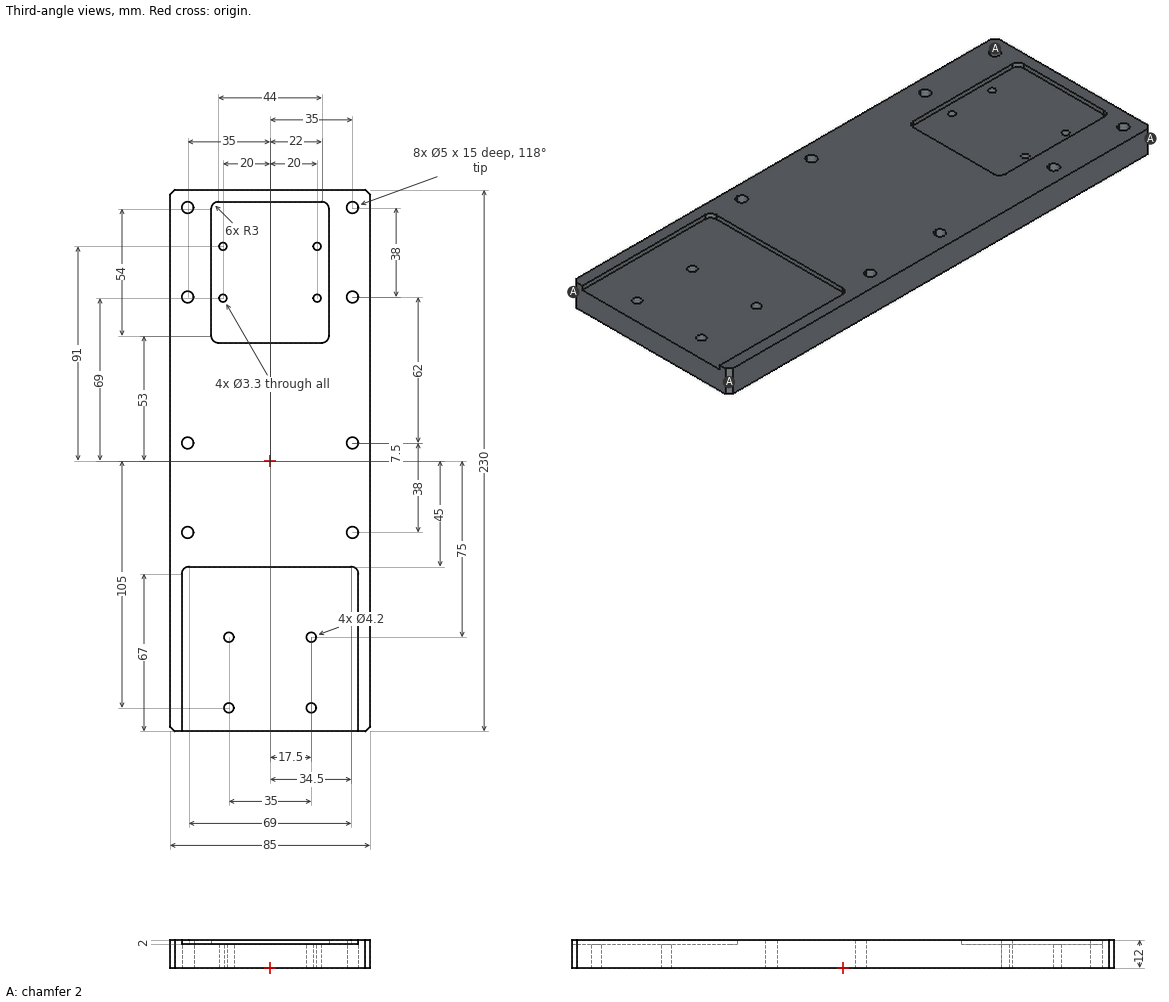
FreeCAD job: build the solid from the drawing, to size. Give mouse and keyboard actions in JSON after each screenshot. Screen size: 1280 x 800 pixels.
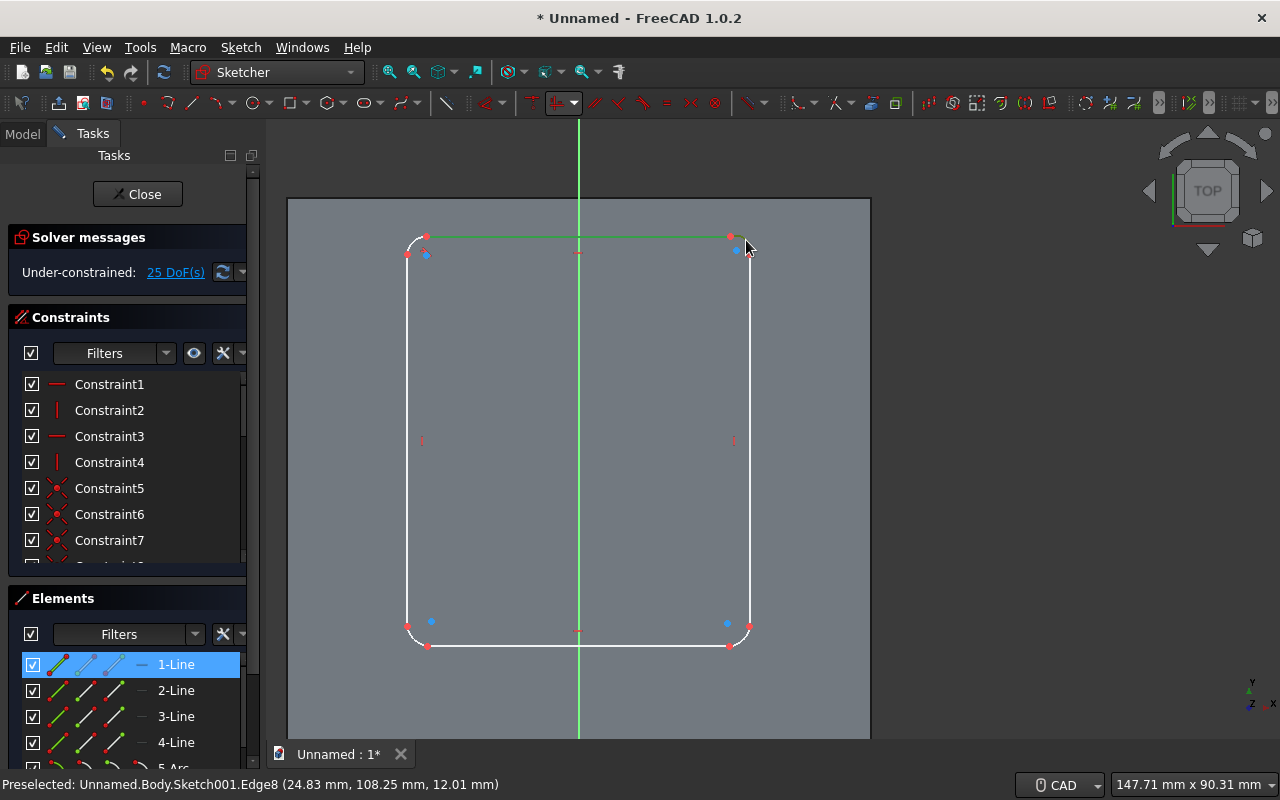
{"action": "key", "text": "t"}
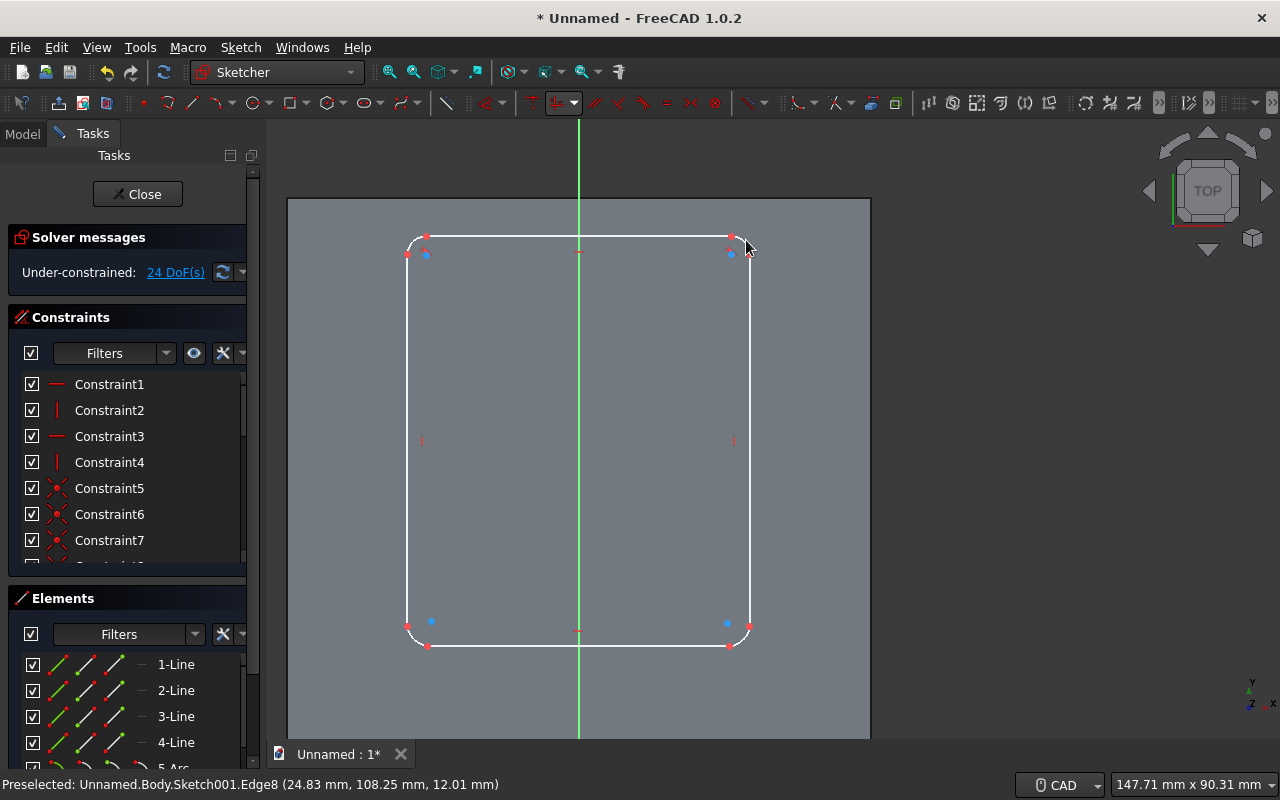
{"action": "scroll", "coordinate": [746, 241], "scroll_direction": "down", "scroll_amount": 7}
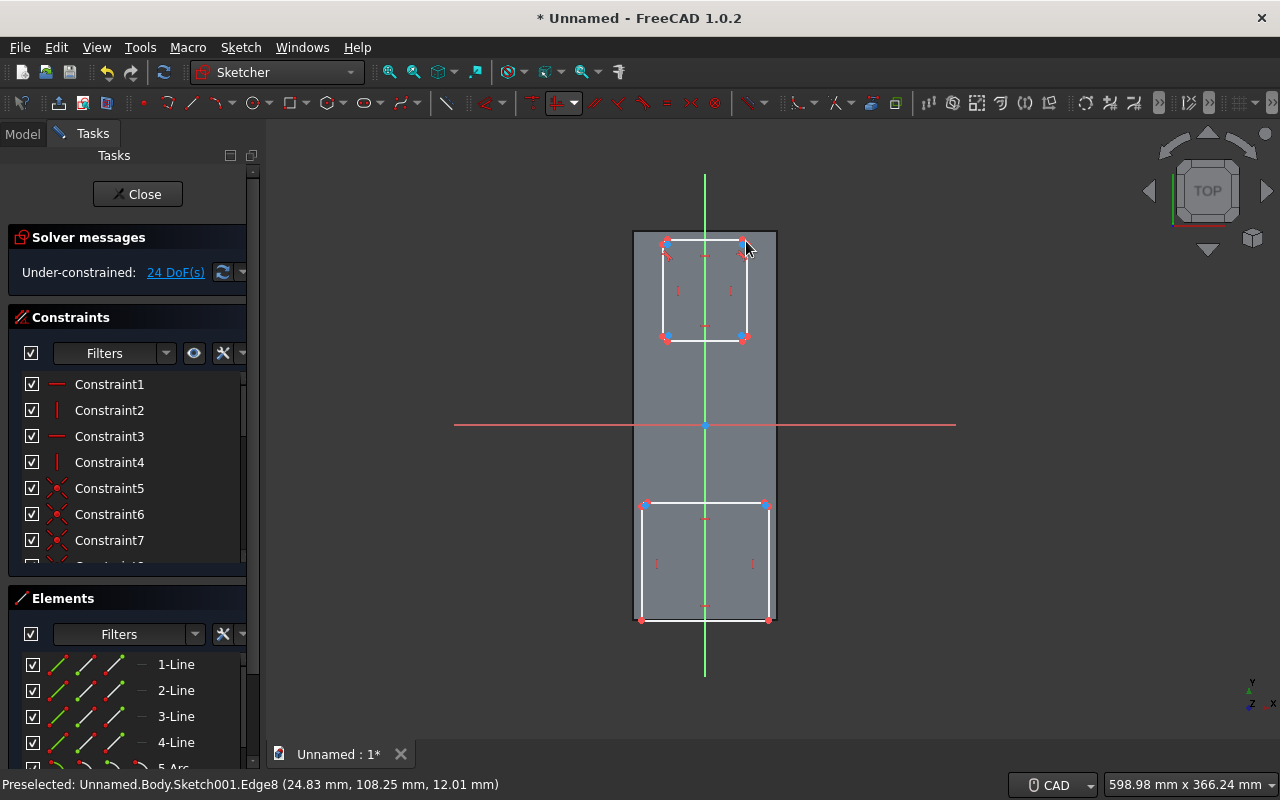
{"action": "left_click", "coordinate": [663, 272]}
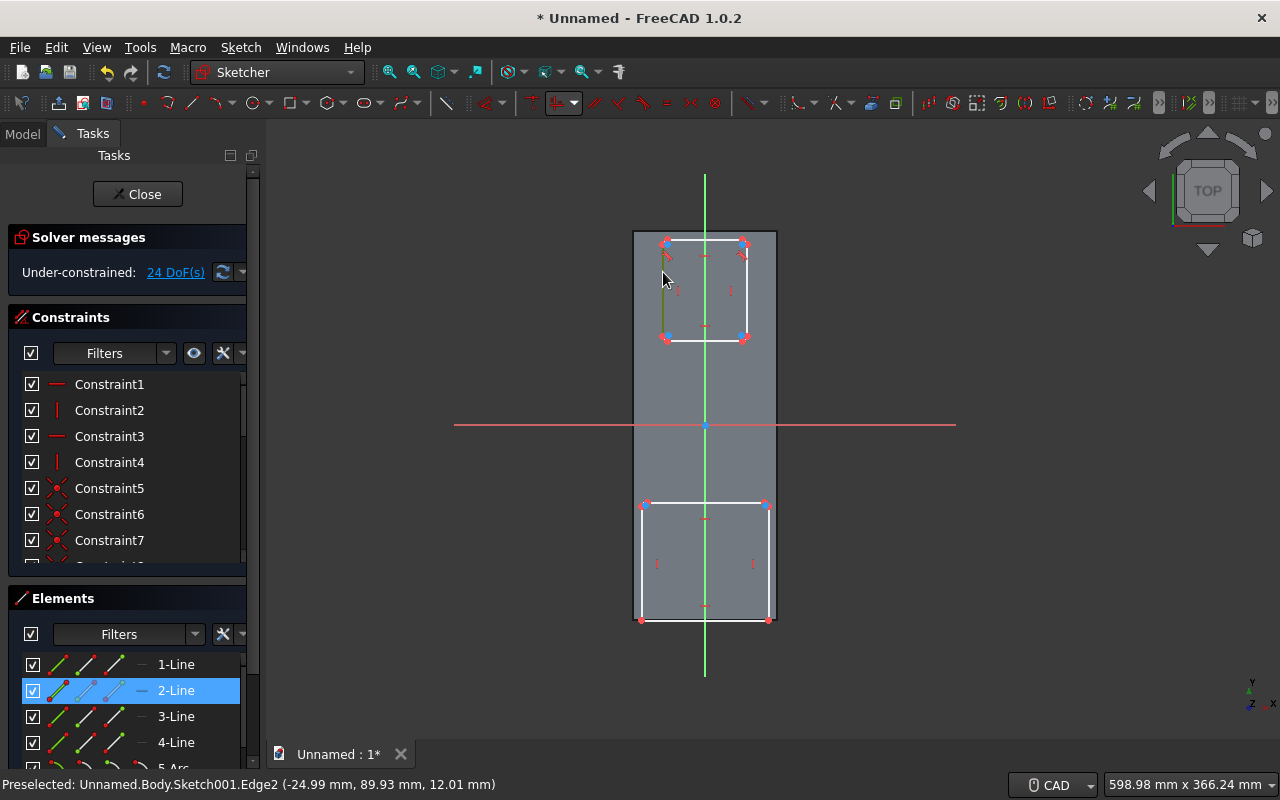
{"action": "scroll", "coordinate": [664, 241], "scroll_direction": "up", "scroll_amount": 7}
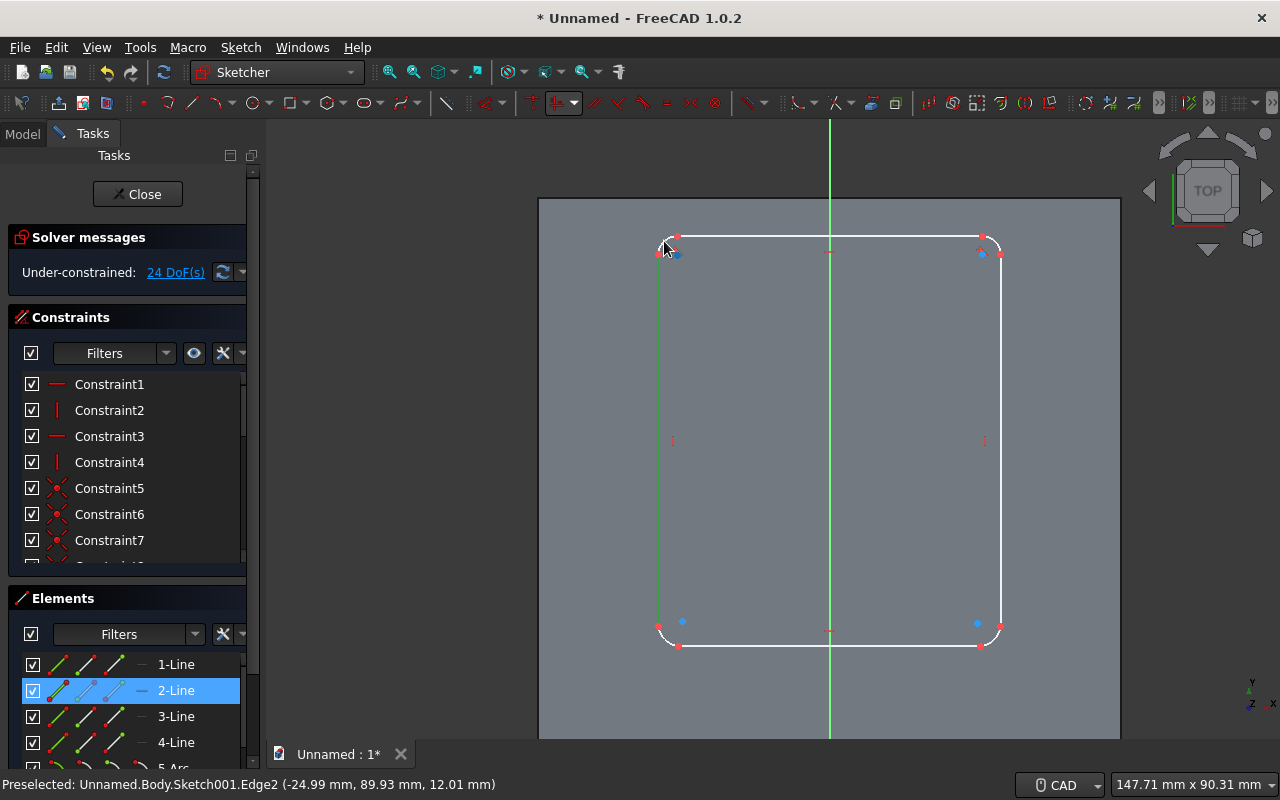
{"action": "left_click", "coordinate": [664, 241]}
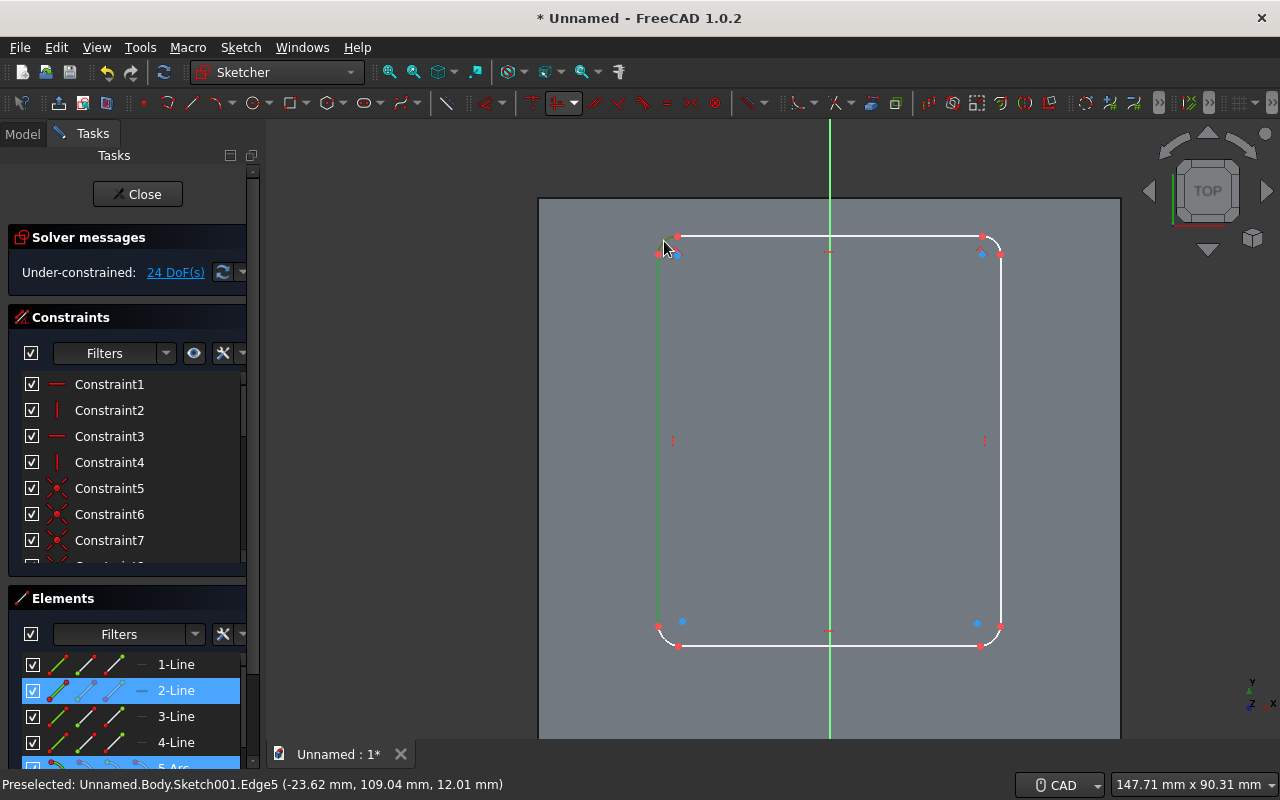
{"action": "key", "text": "t"}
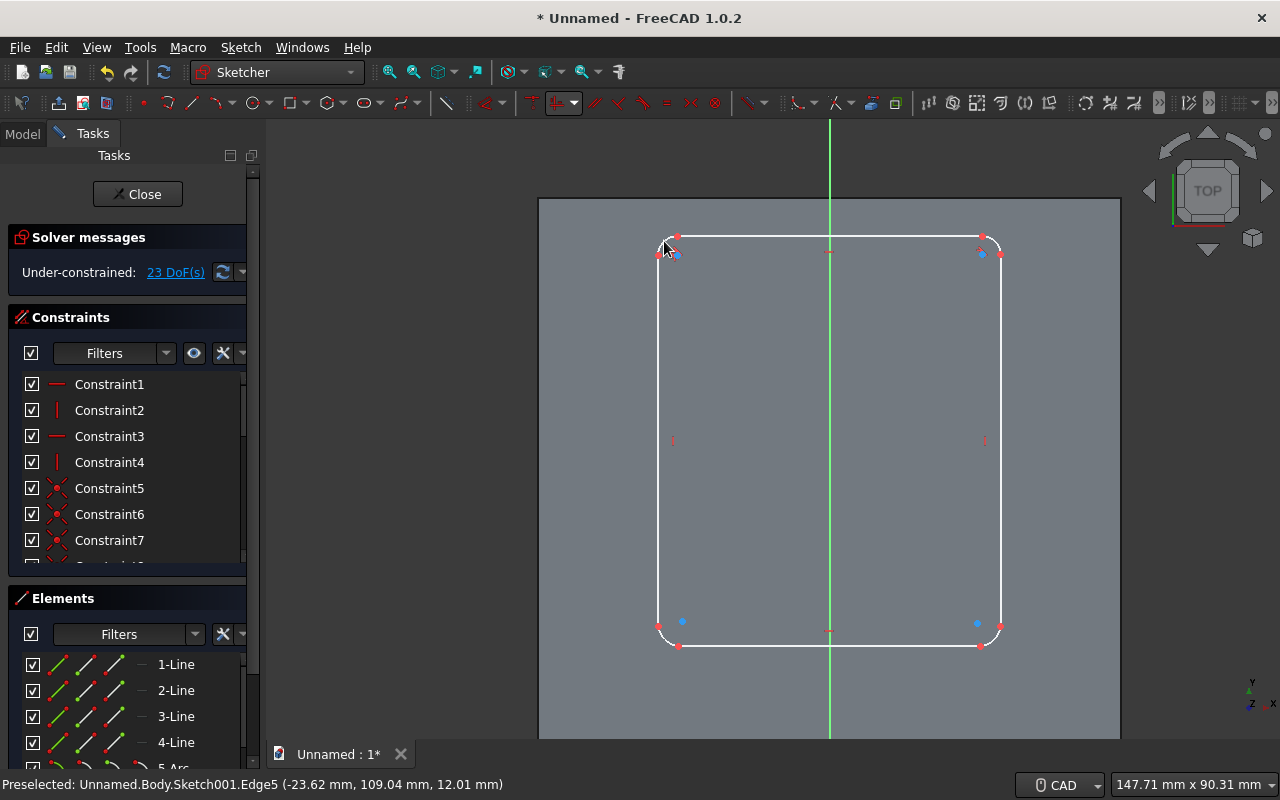
{"action": "scroll", "coordinate": [664, 241], "scroll_direction": "down", "scroll_amount": 7}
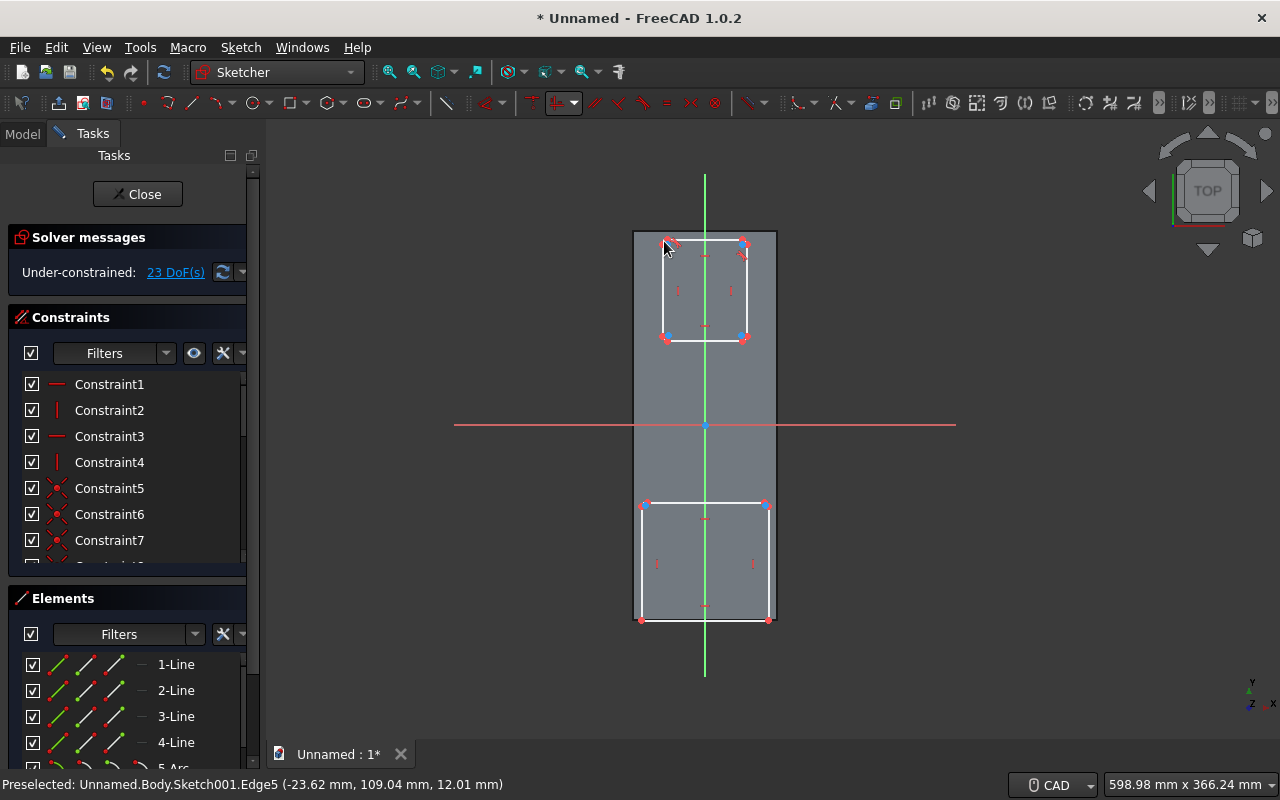
{"action": "left_click", "coordinate": [663, 272]}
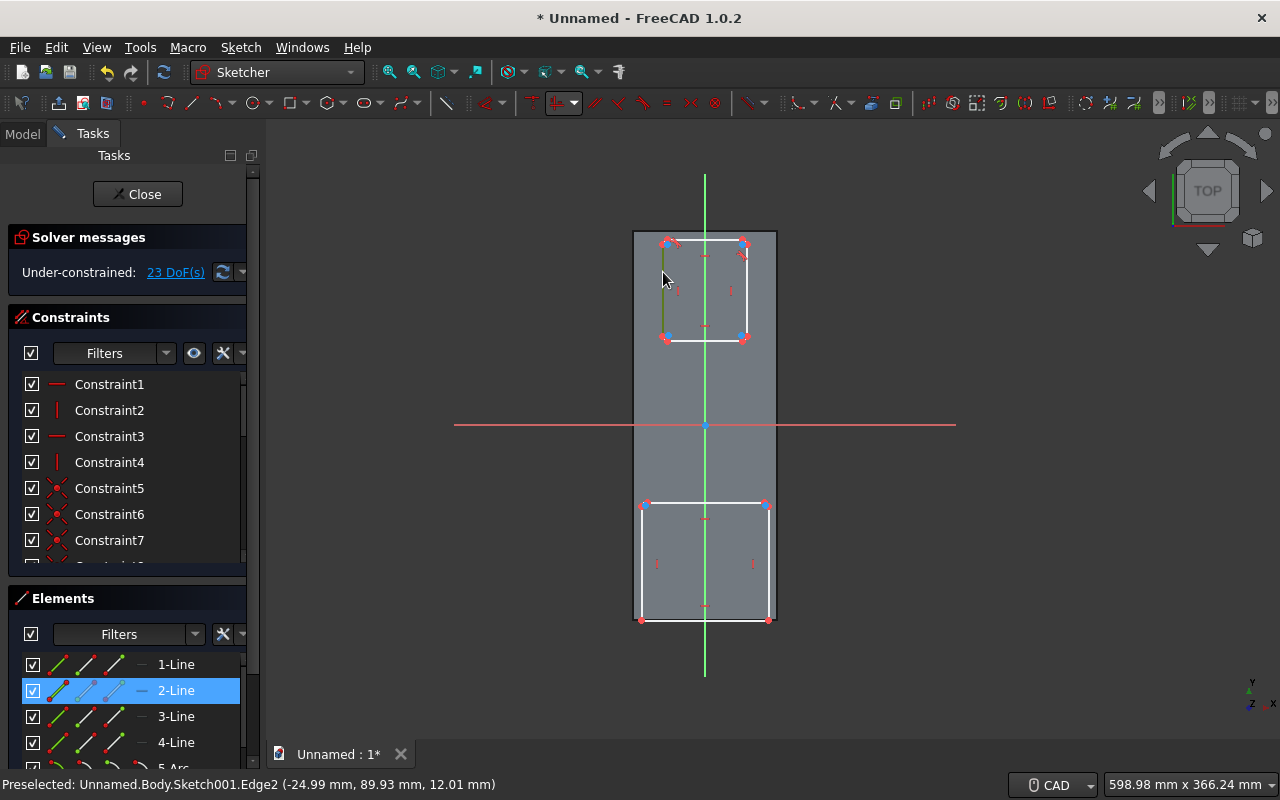
{"action": "scroll", "coordinate": [665, 339], "scroll_direction": "up", "scroll_amount": 7}